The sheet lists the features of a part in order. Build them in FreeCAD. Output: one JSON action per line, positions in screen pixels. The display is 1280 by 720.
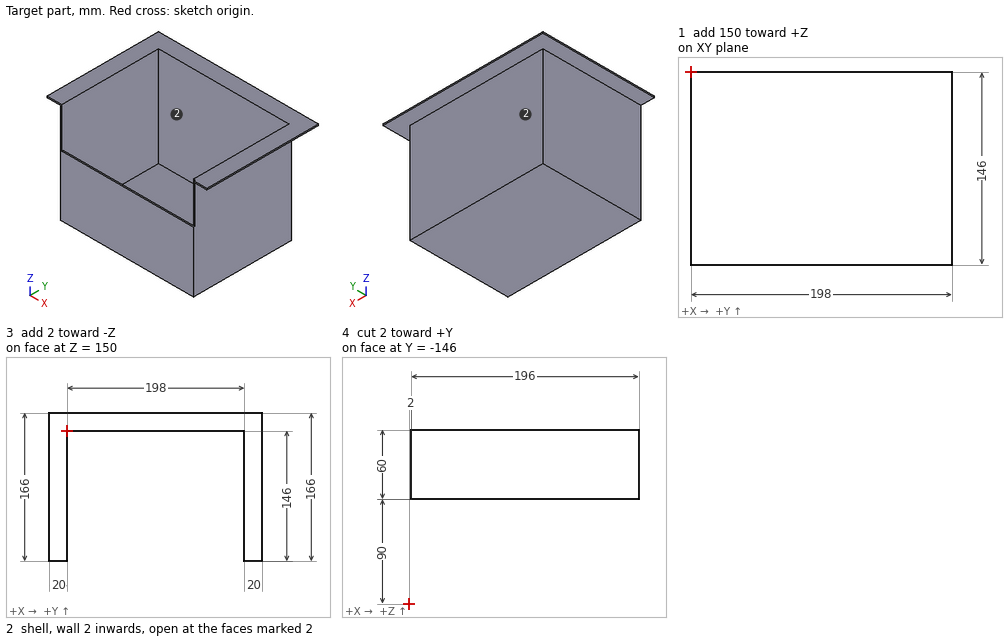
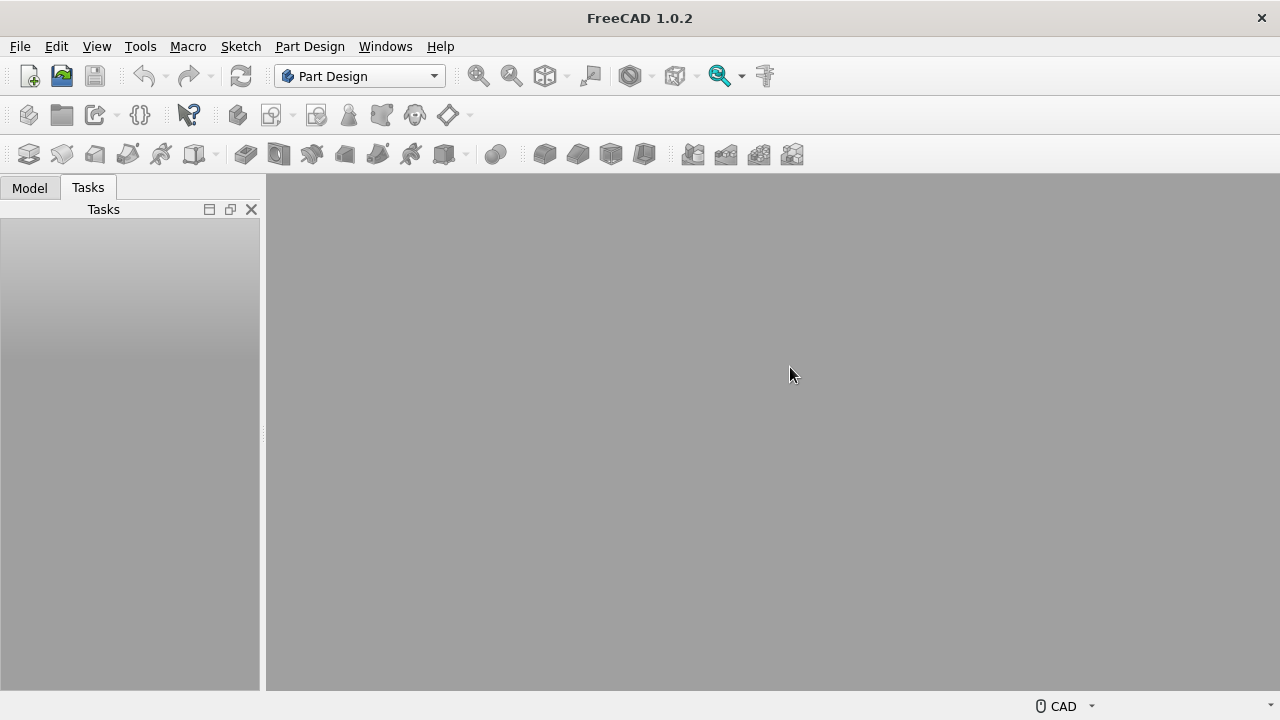
{"action": "left_click", "coordinate": [29, 76]}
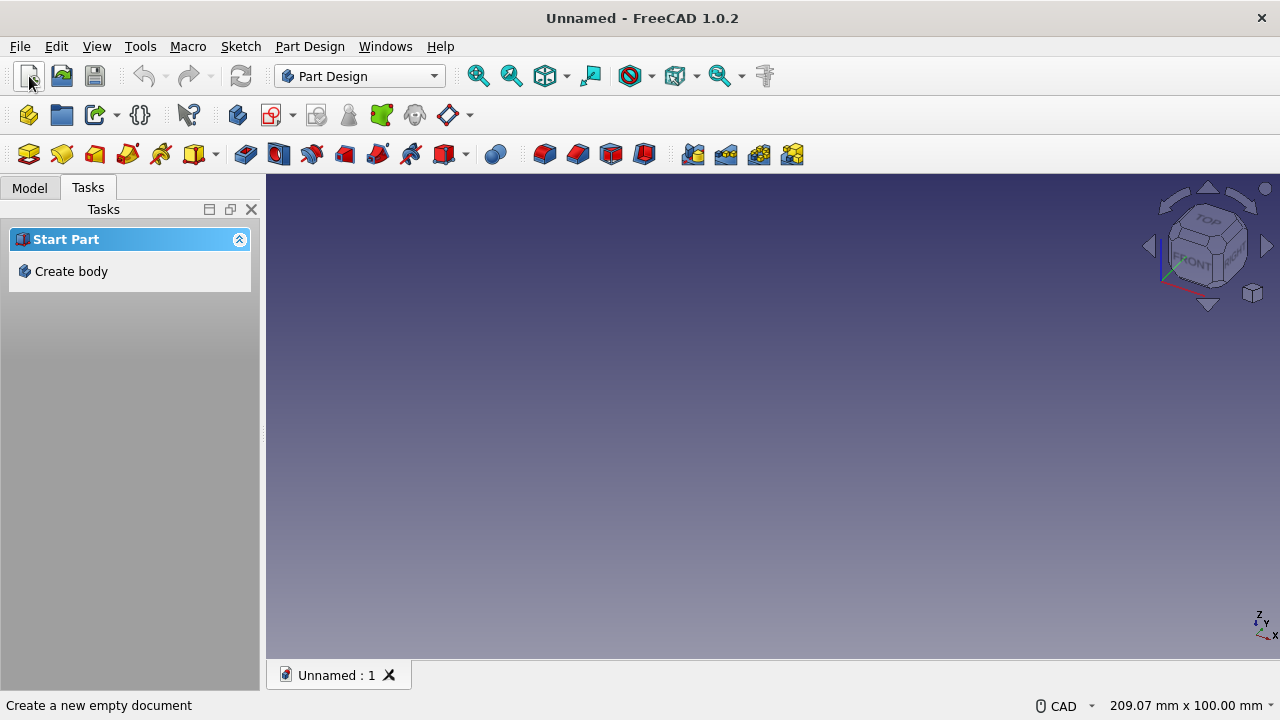
{"action": "left_click", "coordinate": [270, 116]}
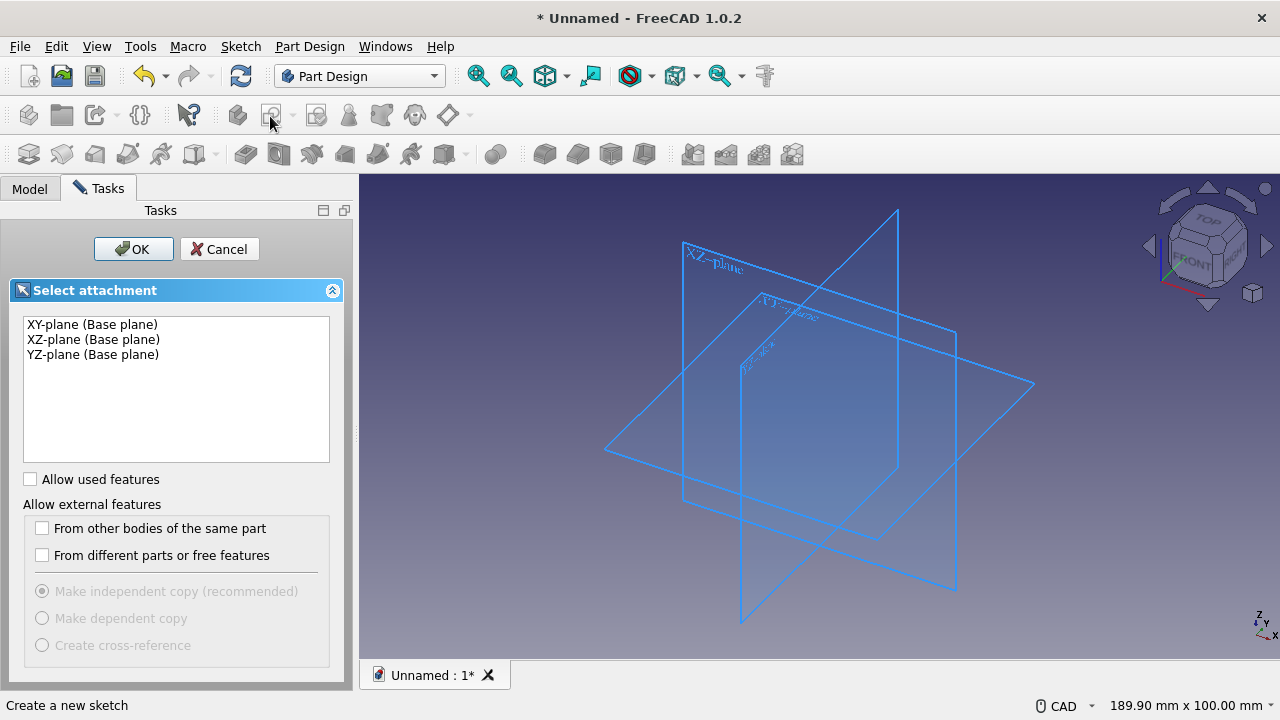
{"action": "left_click", "coordinate": [84, 324]}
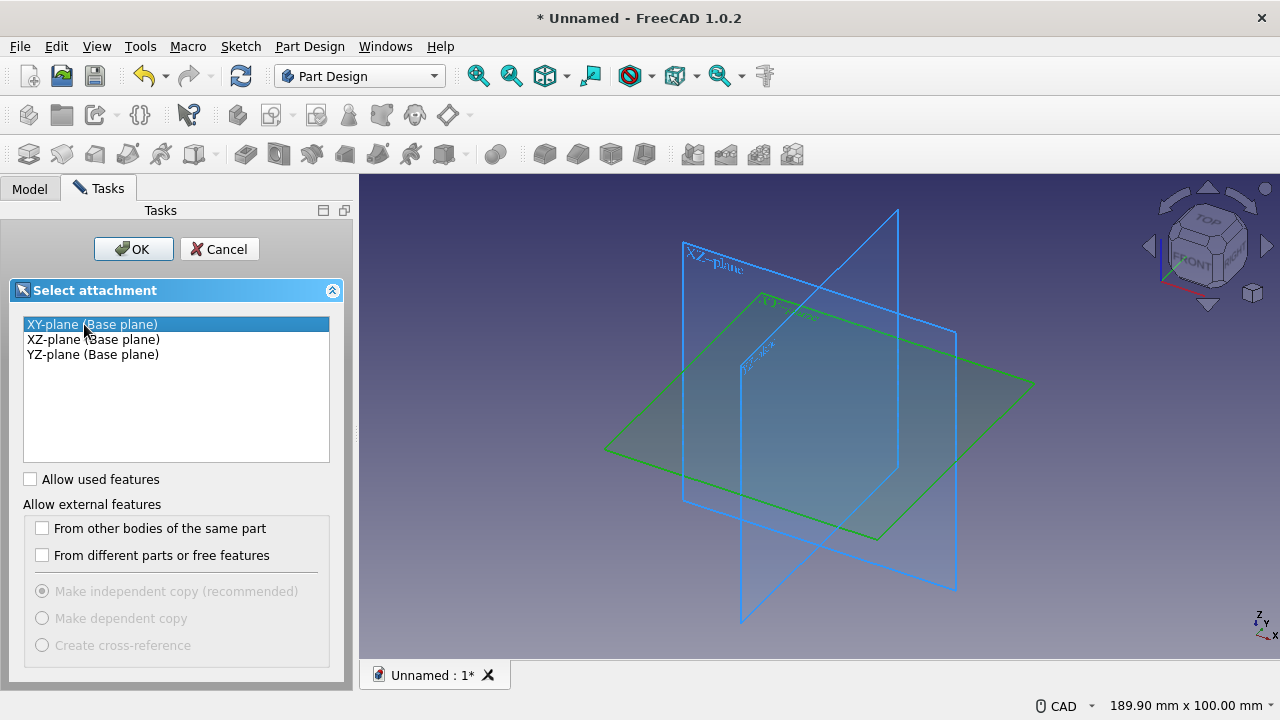
{"action": "left_click", "coordinate": [134, 249]}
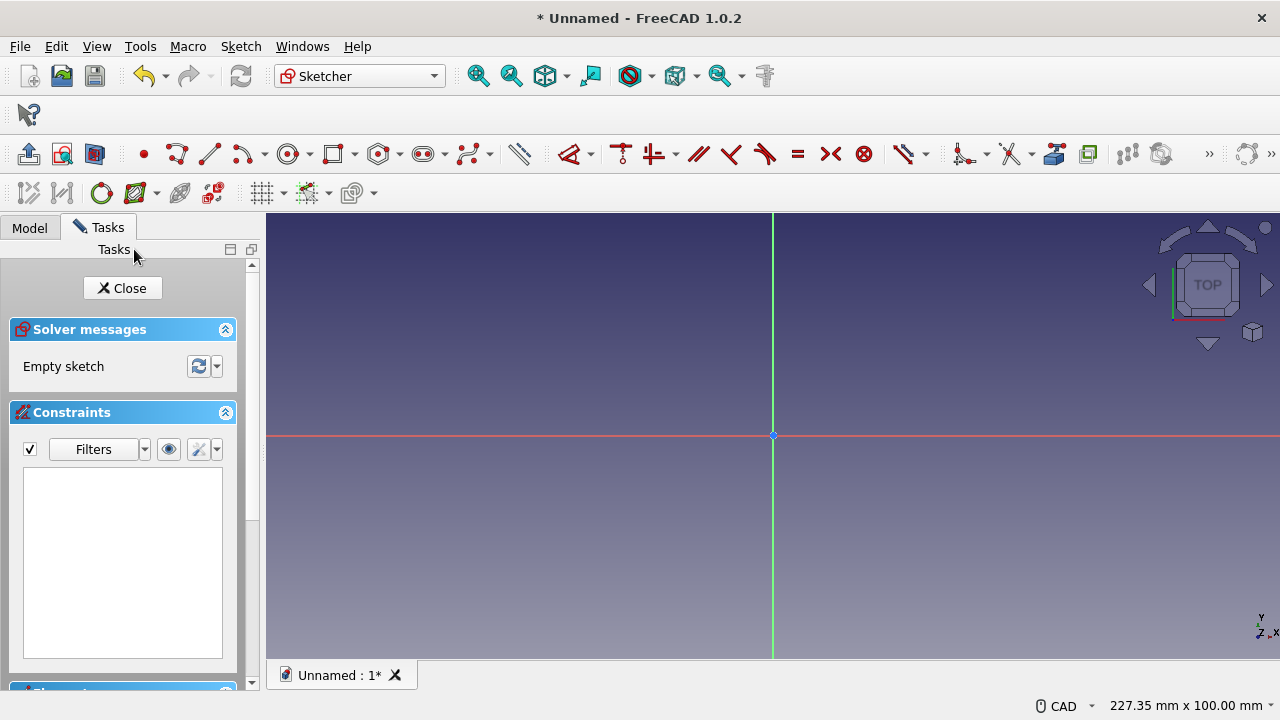
{"action": "scroll", "coordinate": [408, 247], "scroll_direction": "down", "scroll_amount": 5}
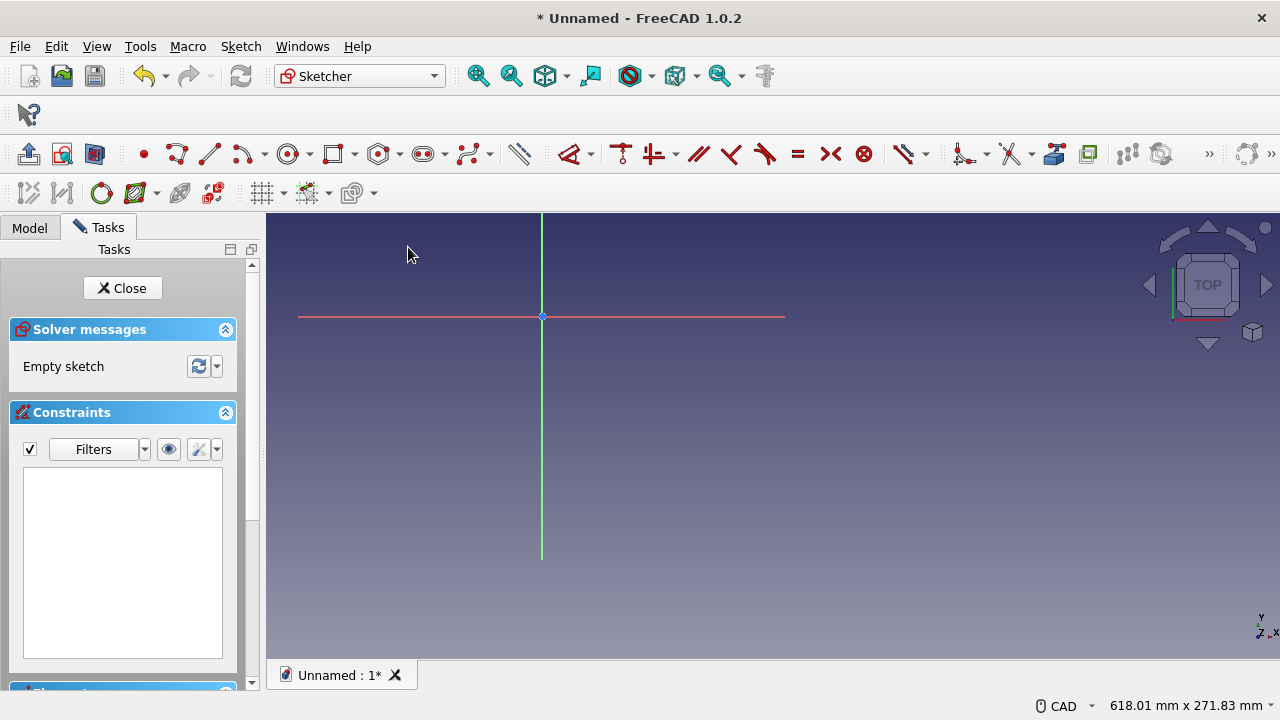
{"action": "left_click", "coordinate": [332, 154]}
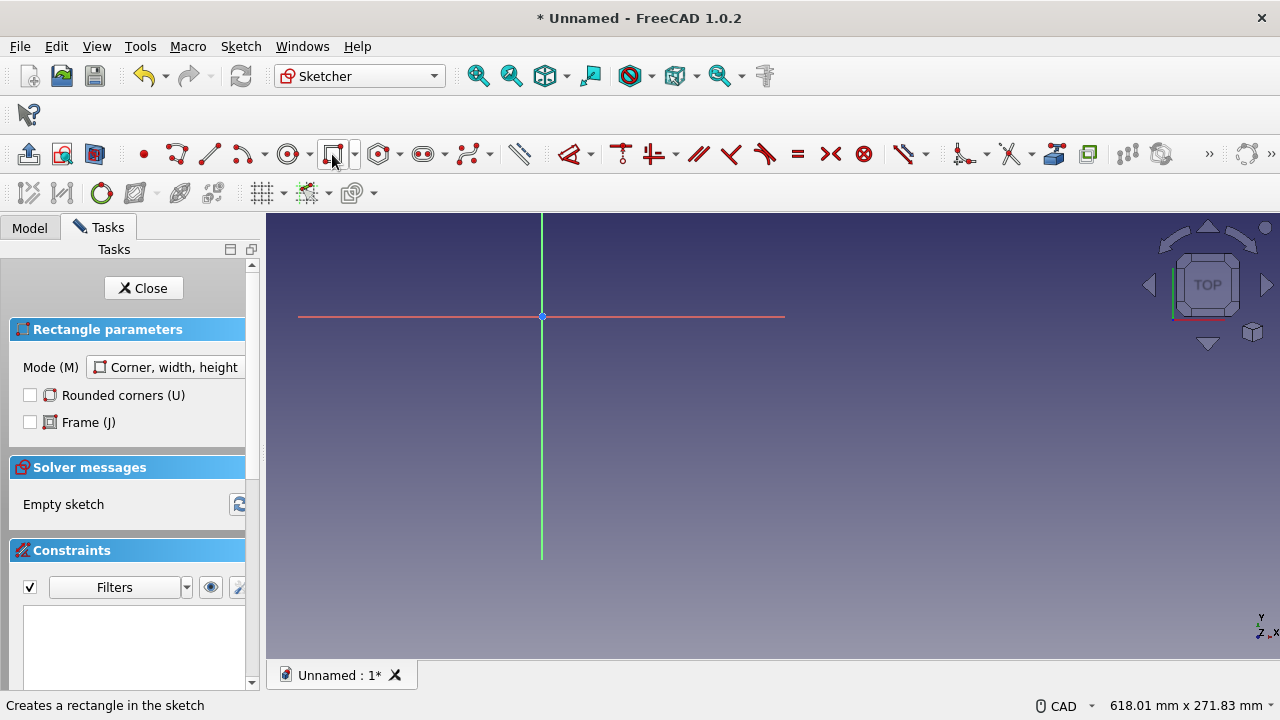
{"action": "left_click", "coordinate": [542, 317]}
{"action": "mouse_move", "coordinate": [867, 556]}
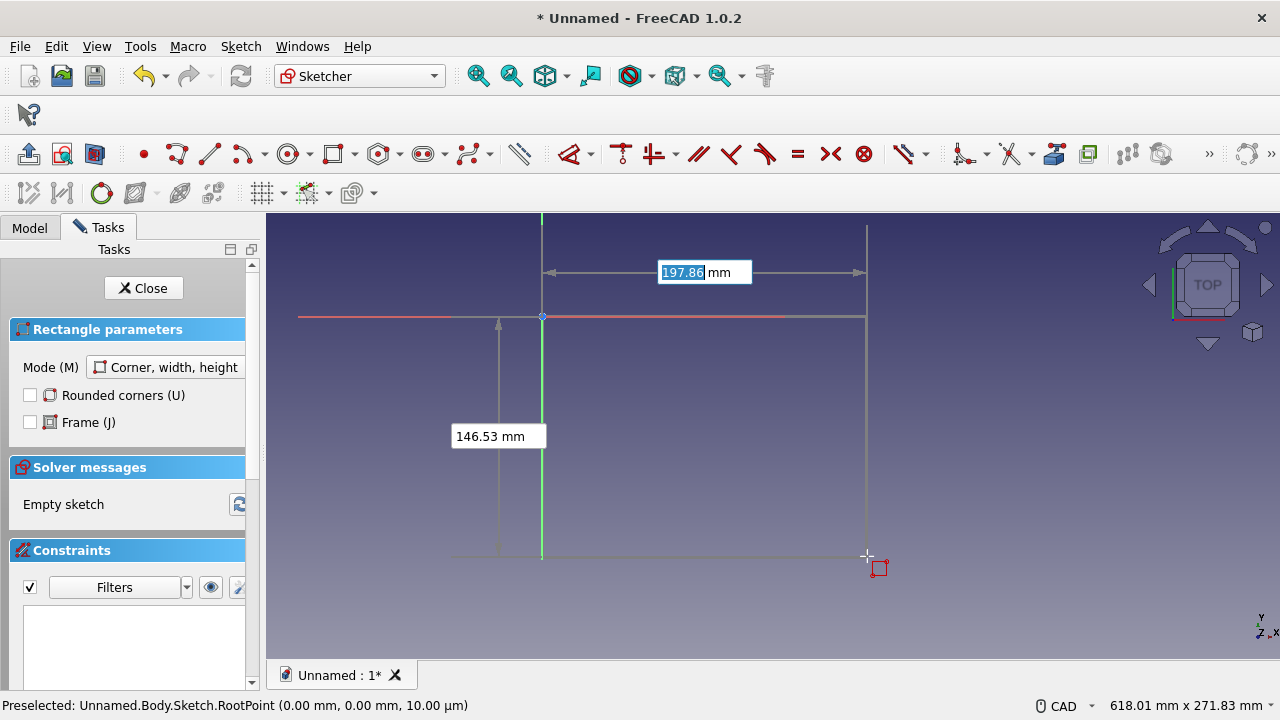
{"action": "type", "text": "198"}
{"action": "key", "text": "Tab"}
{"action": "type", "text": "146"}
{"action": "key", "text": "Return"}
{"action": "key", "text": "Escape"}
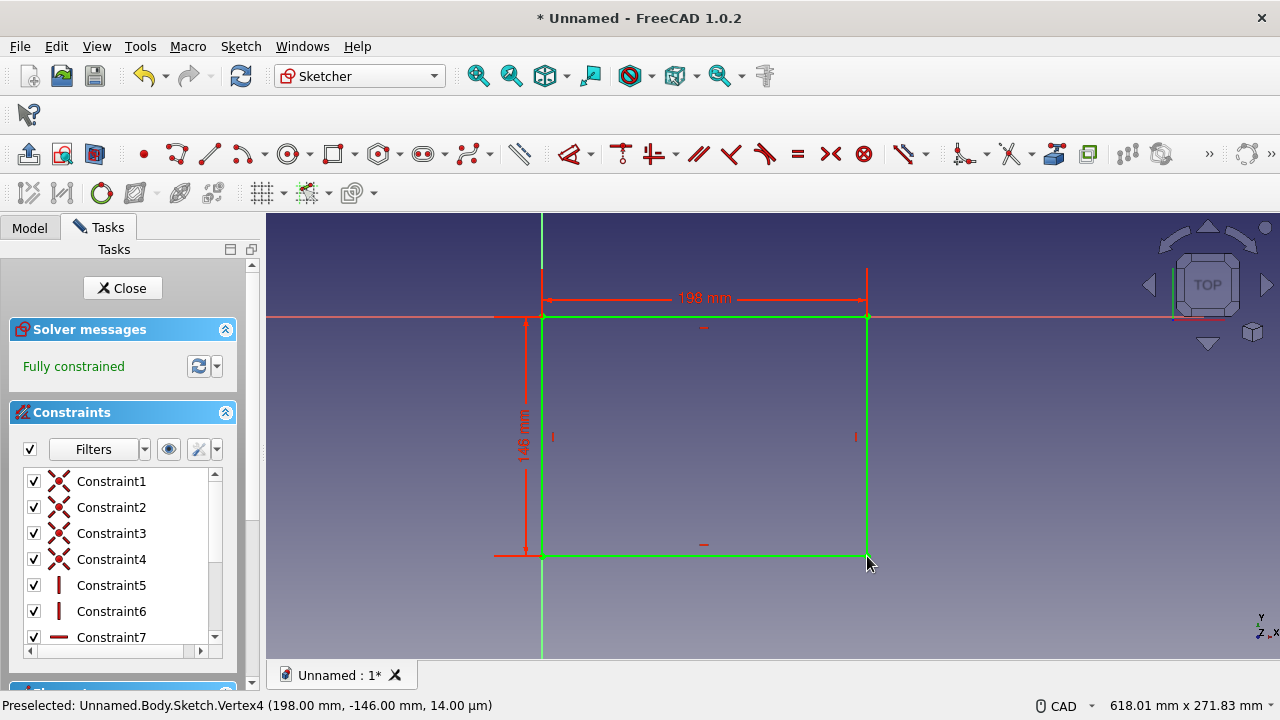
{"action": "left_click", "coordinate": [123, 288]}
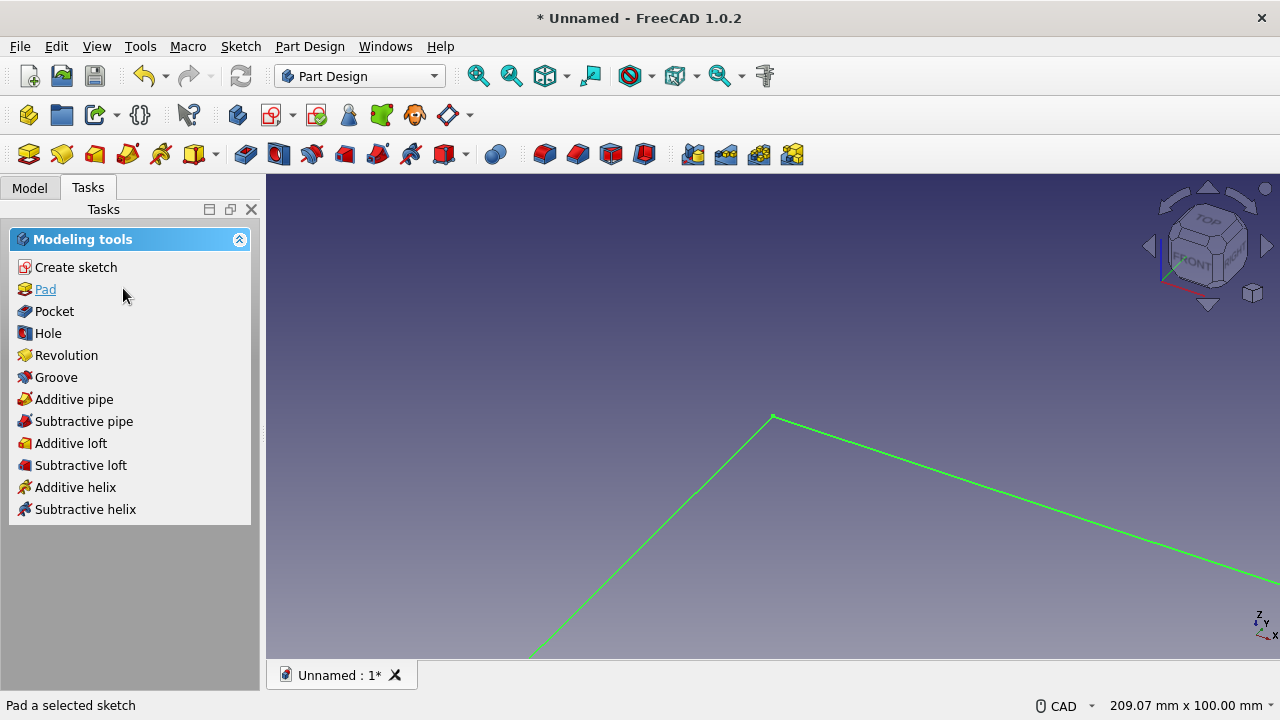
{"action": "left_click", "coordinate": [29, 154]}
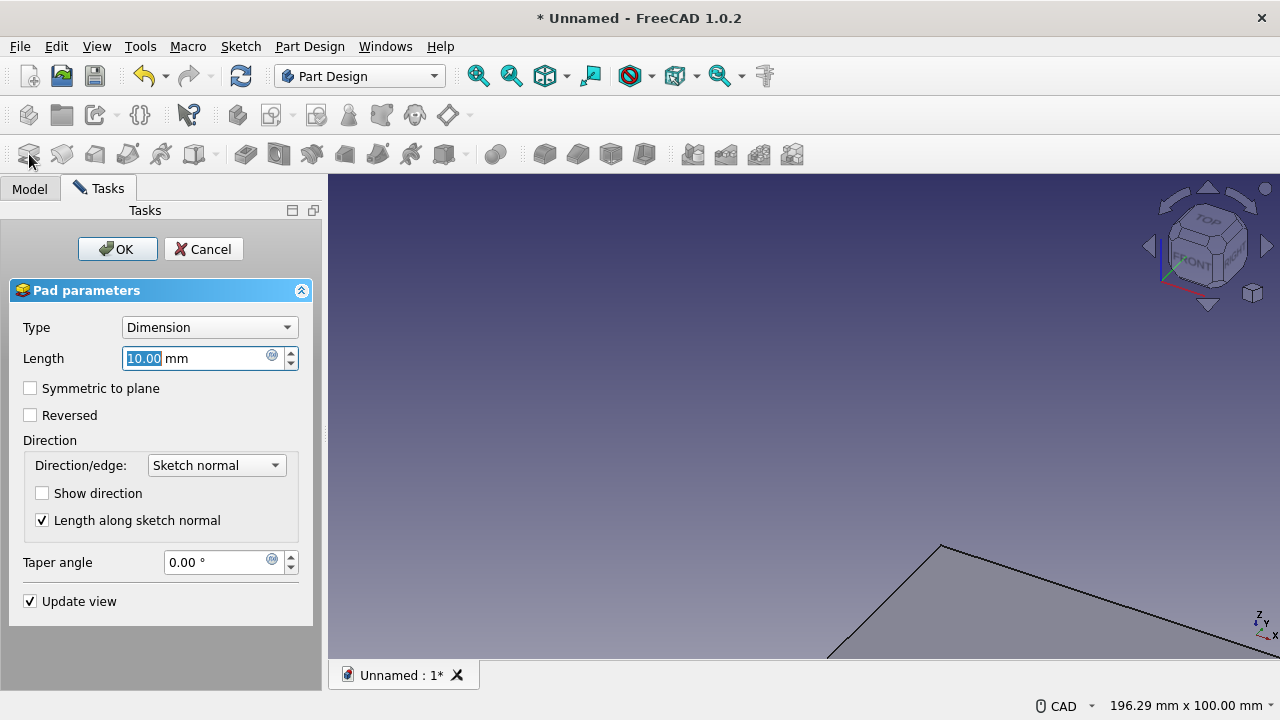
{"action": "type", "text": "150"}
{"action": "key", "text": "Tab"}